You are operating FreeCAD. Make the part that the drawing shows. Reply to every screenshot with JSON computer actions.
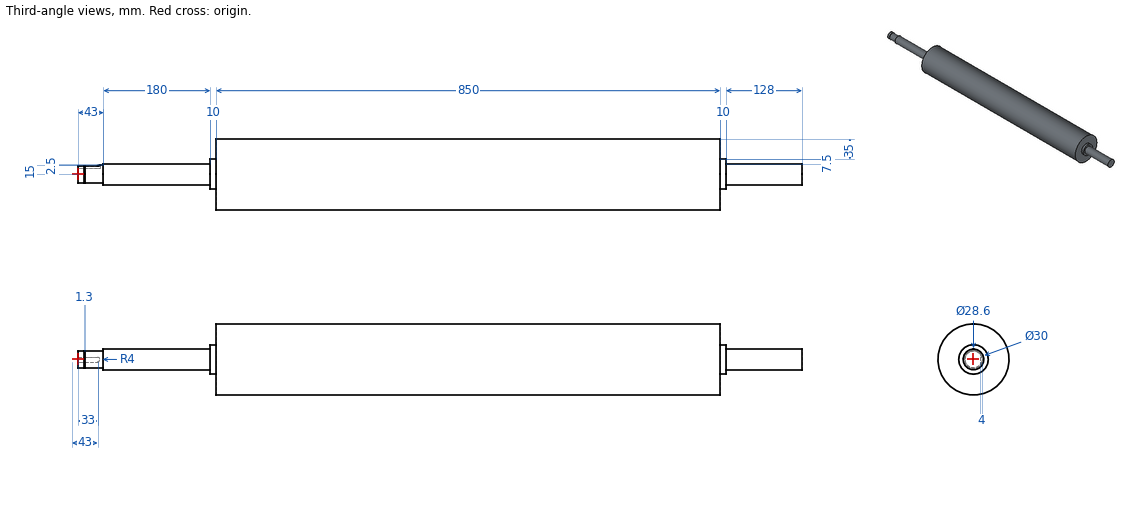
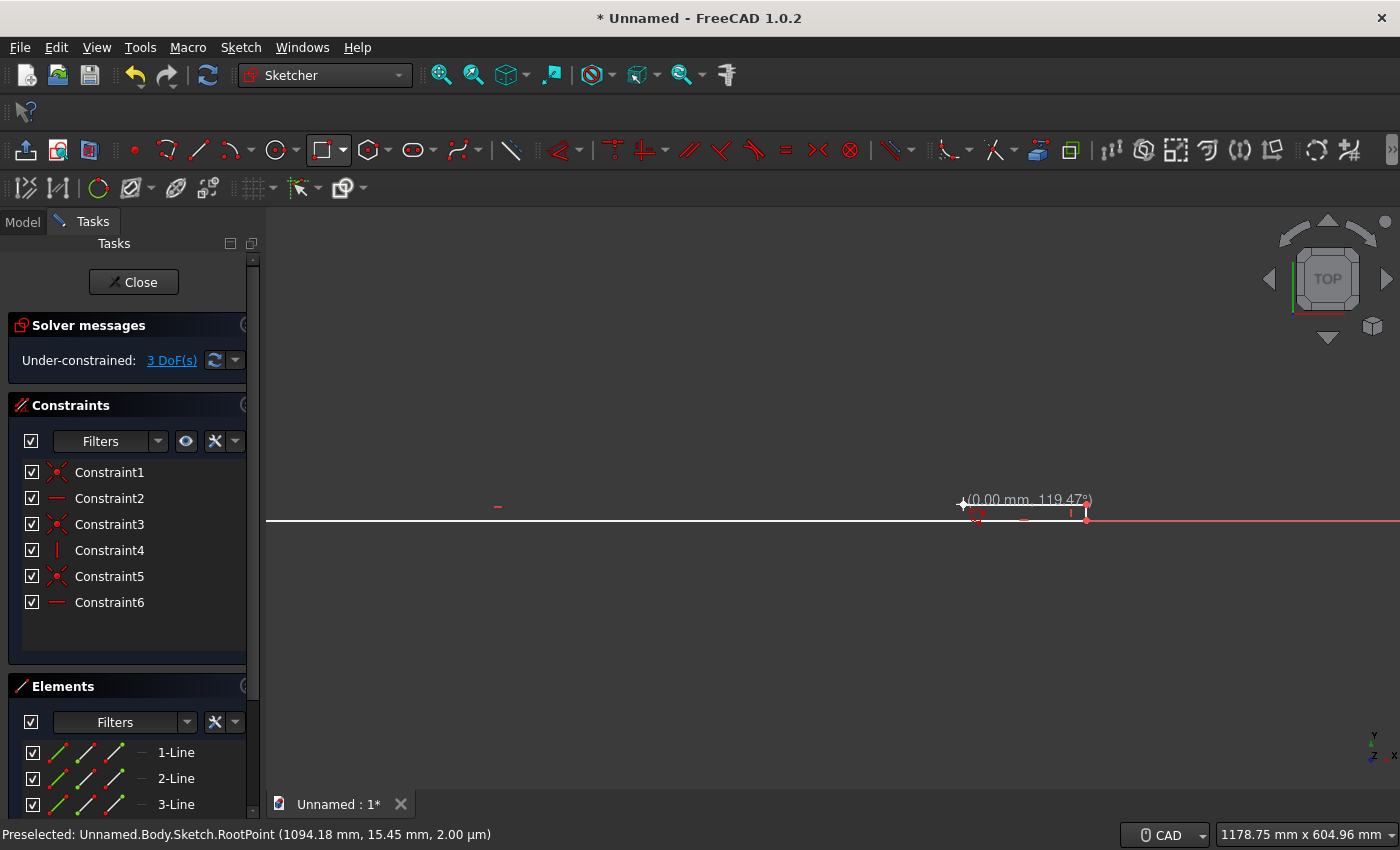
{"action": "scroll", "coordinate": [963, 497], "scroll_direction": "up", "scroll_amount": 4}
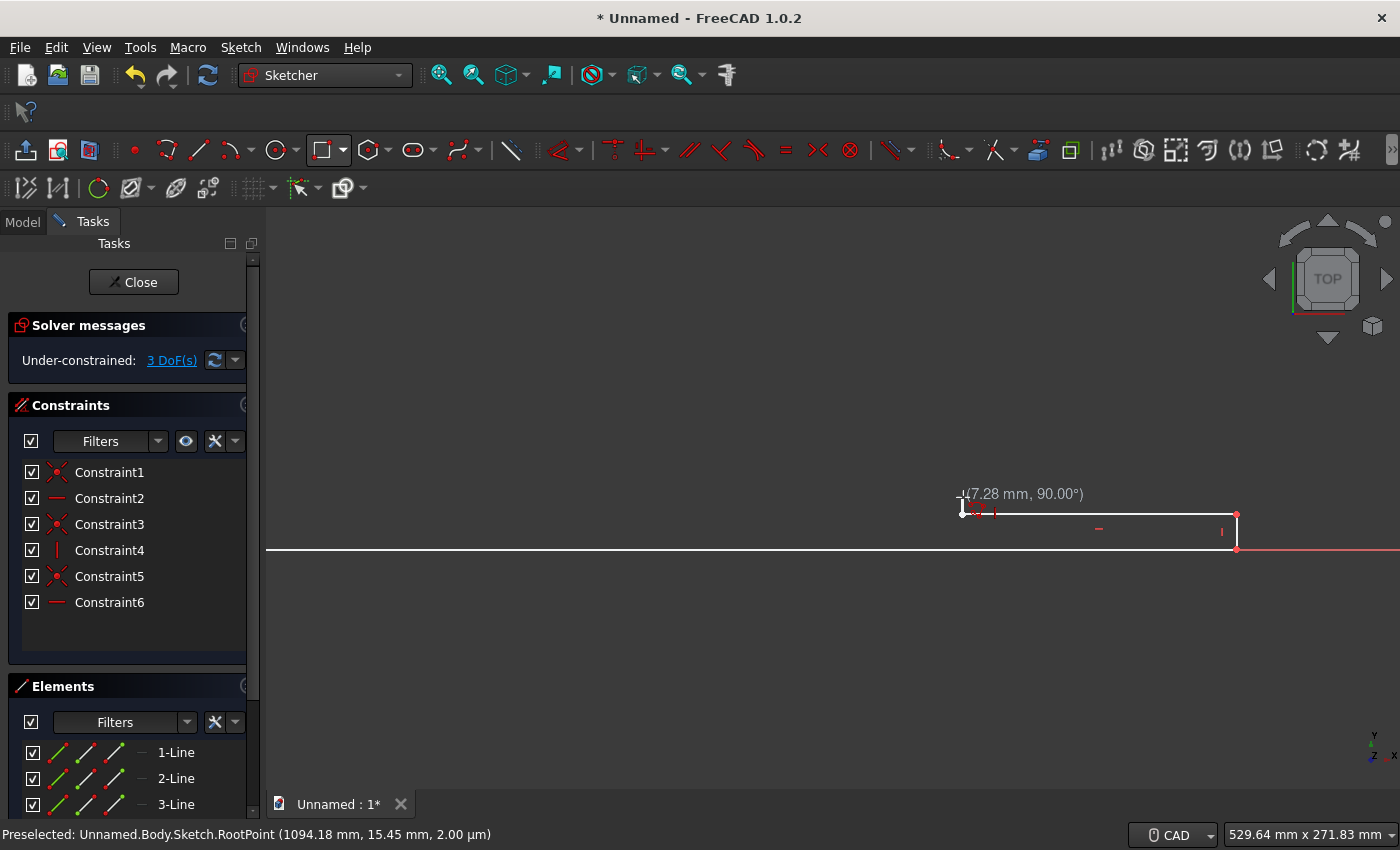
{"action": "left_click", "coordinate": [962, 496]}
{"action": "left_click", "coordinate": [941, 496]}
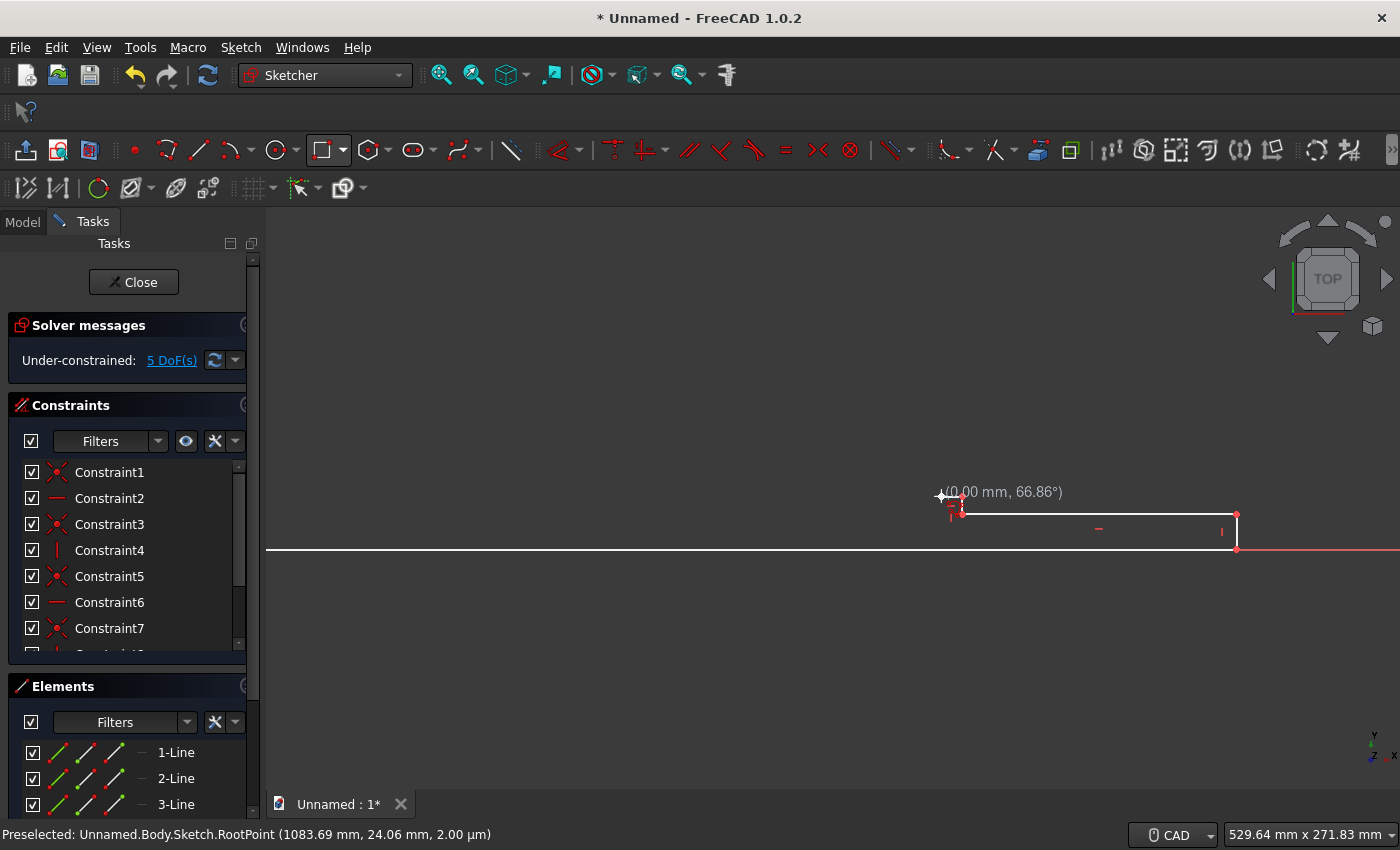
{"action": "scroll", "coordinate": [1038, 502], "scroll_direction": "down", "scroll_amount": 7}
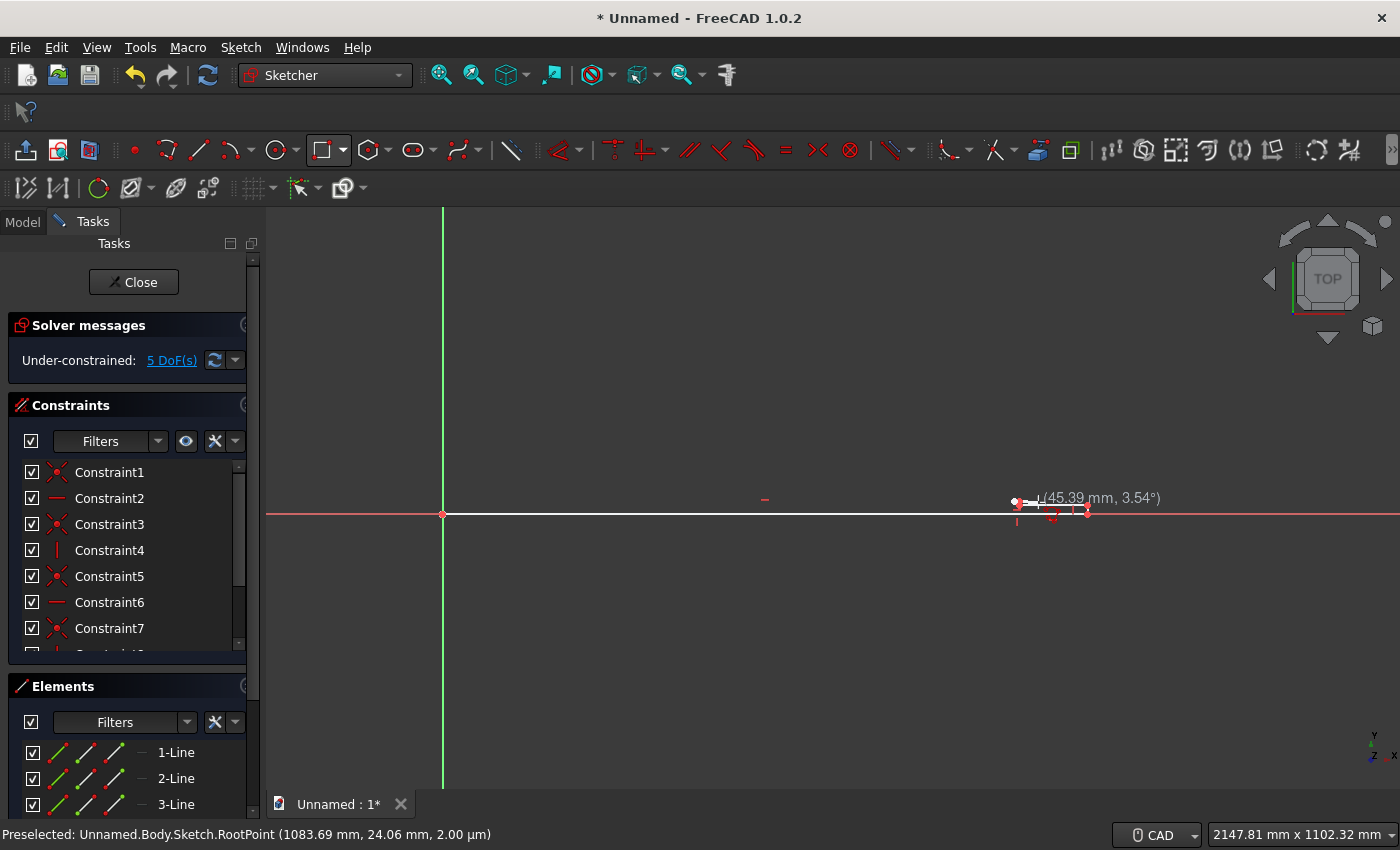
{"action": "left_click", "coordinate": [1015, 482]}
{"action": "left_click", "coordinate": [566, 482]}
{"action": "left_click", "coordinate": [566, 501]}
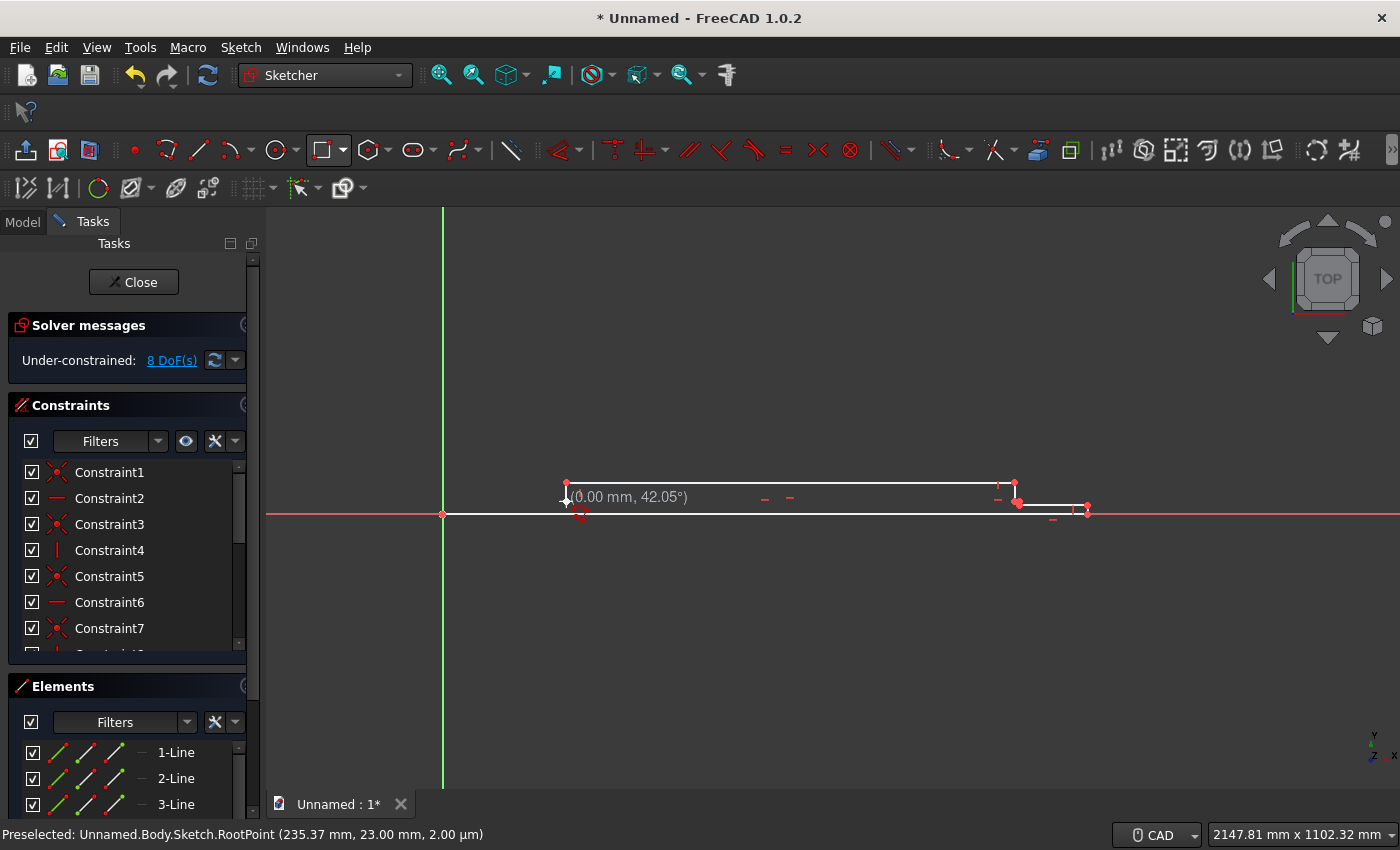
{"action": "scroll", "coordinate": [560, 501], "scroll_direction": "up", "scroll_amount": 6}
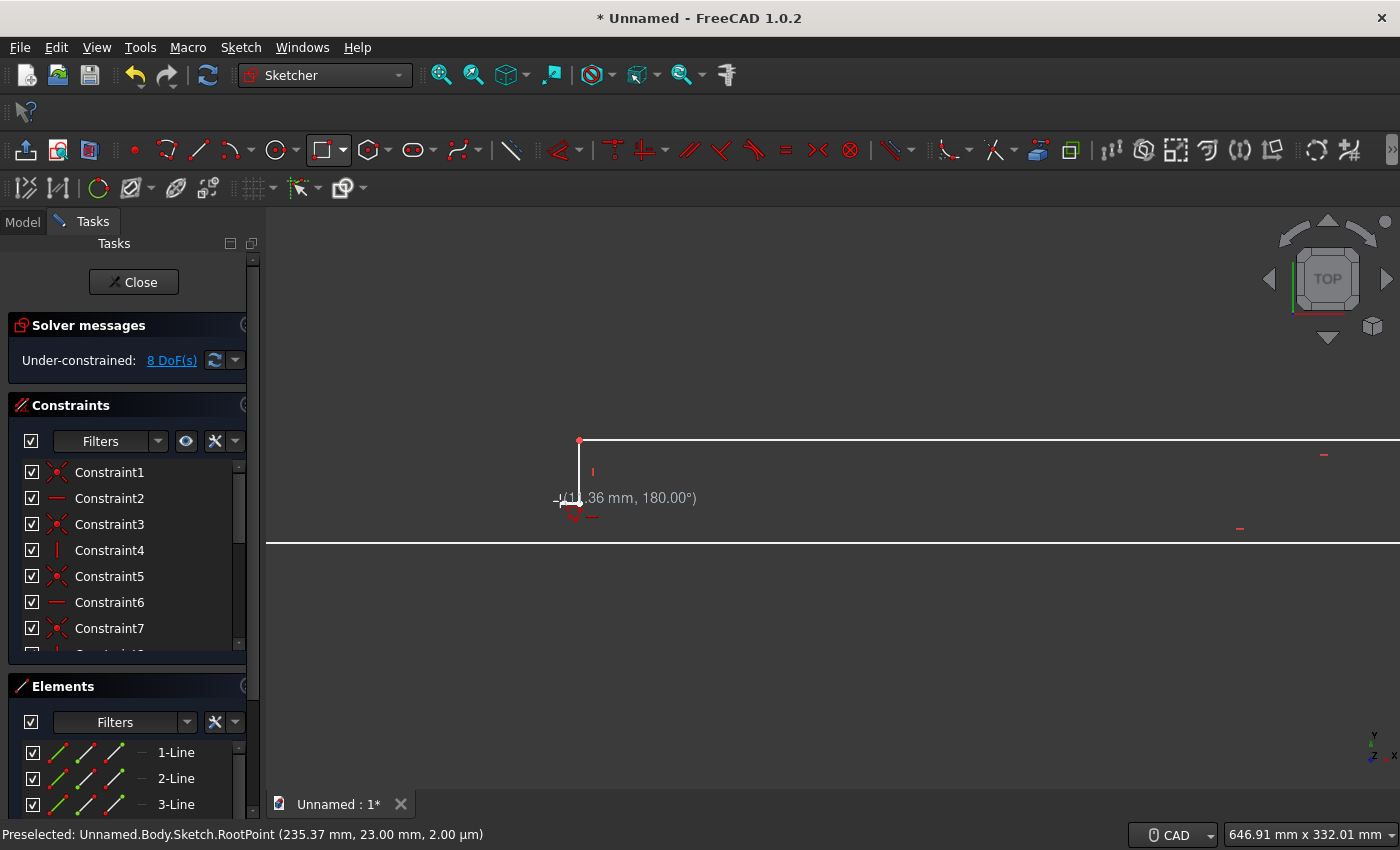
{"action": "left_click", "coordinate": [561, 500]}
{"action": "left_click", "coordinate": [561, 513]}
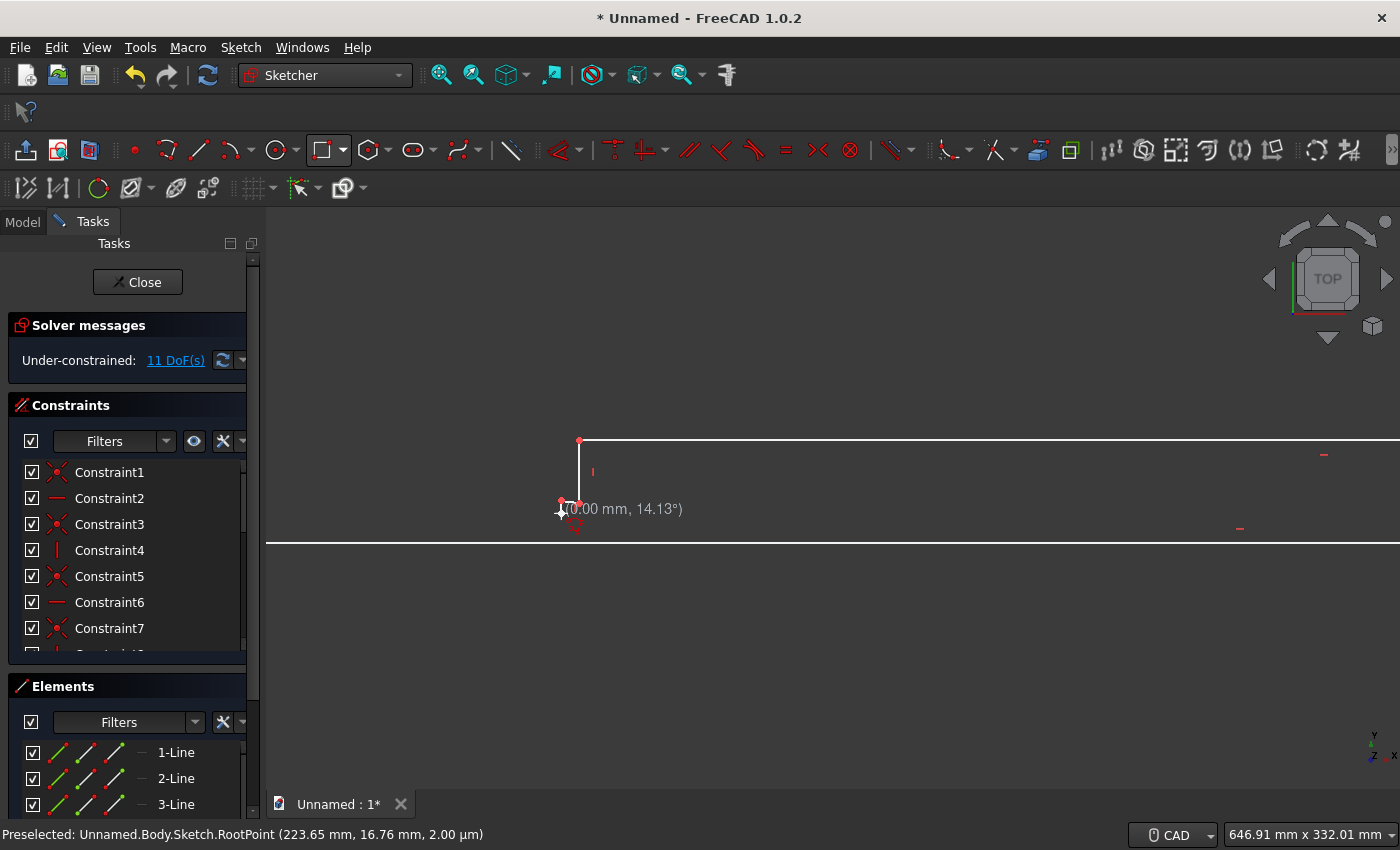
{"action": "scroll", "coordinate": [560, 501], "scroll_direction": "down", "scroll_amount": 6}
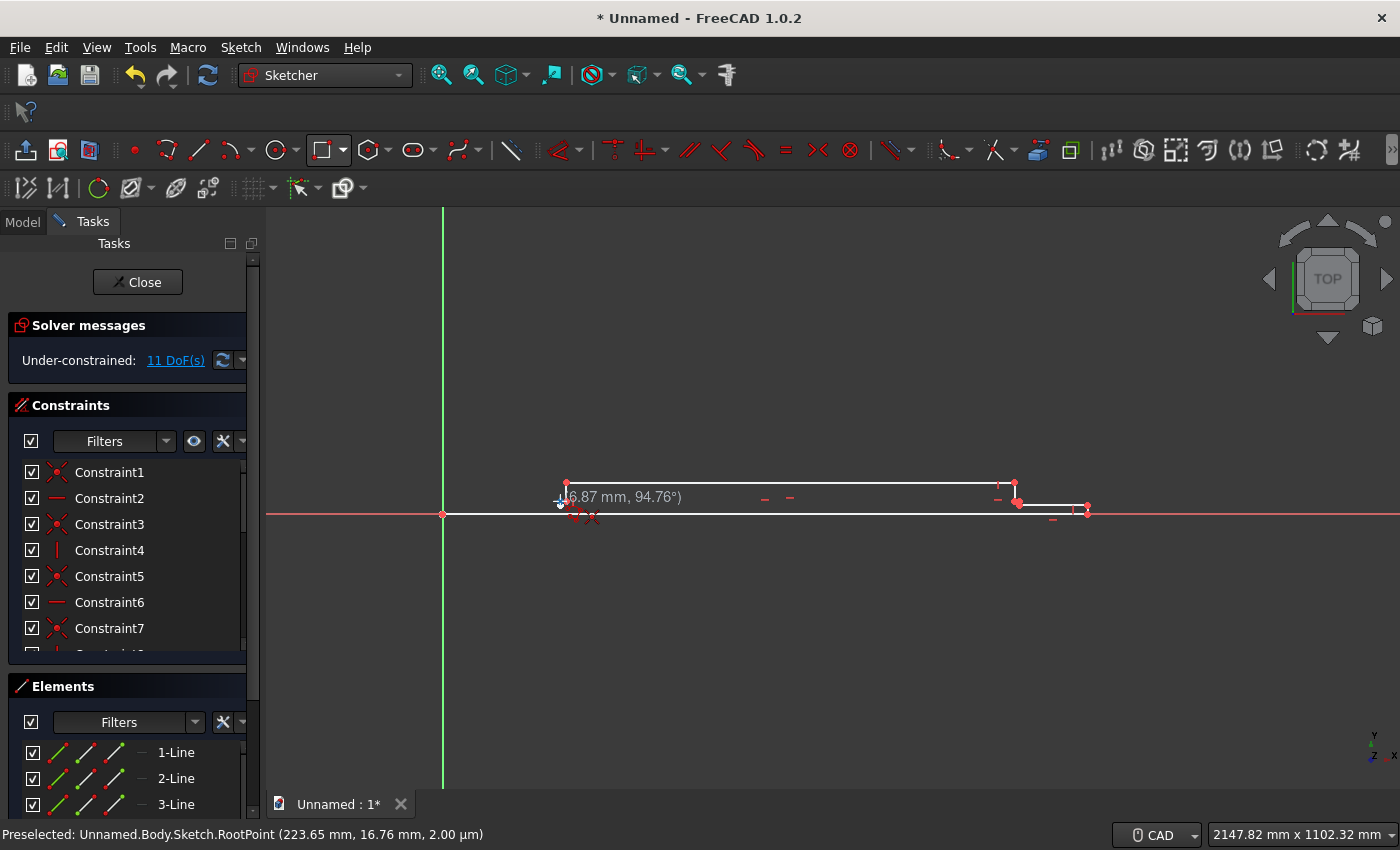
{"action": "scroll", "coordinate": [465, 505], "scroll_direction": "up", "scroll_amount": 3}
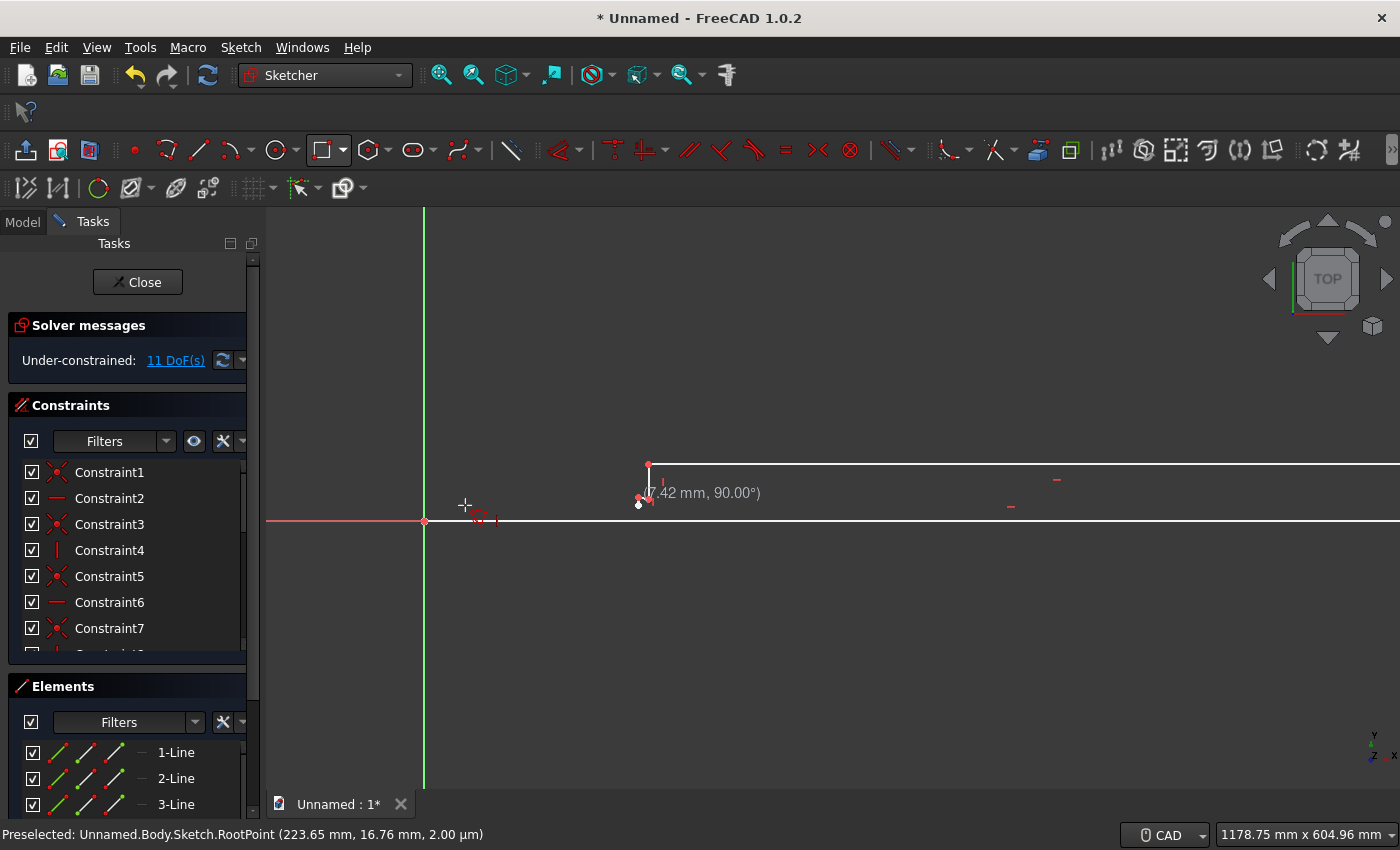
{"action": "left_click", "coordinate": [466, 505]}